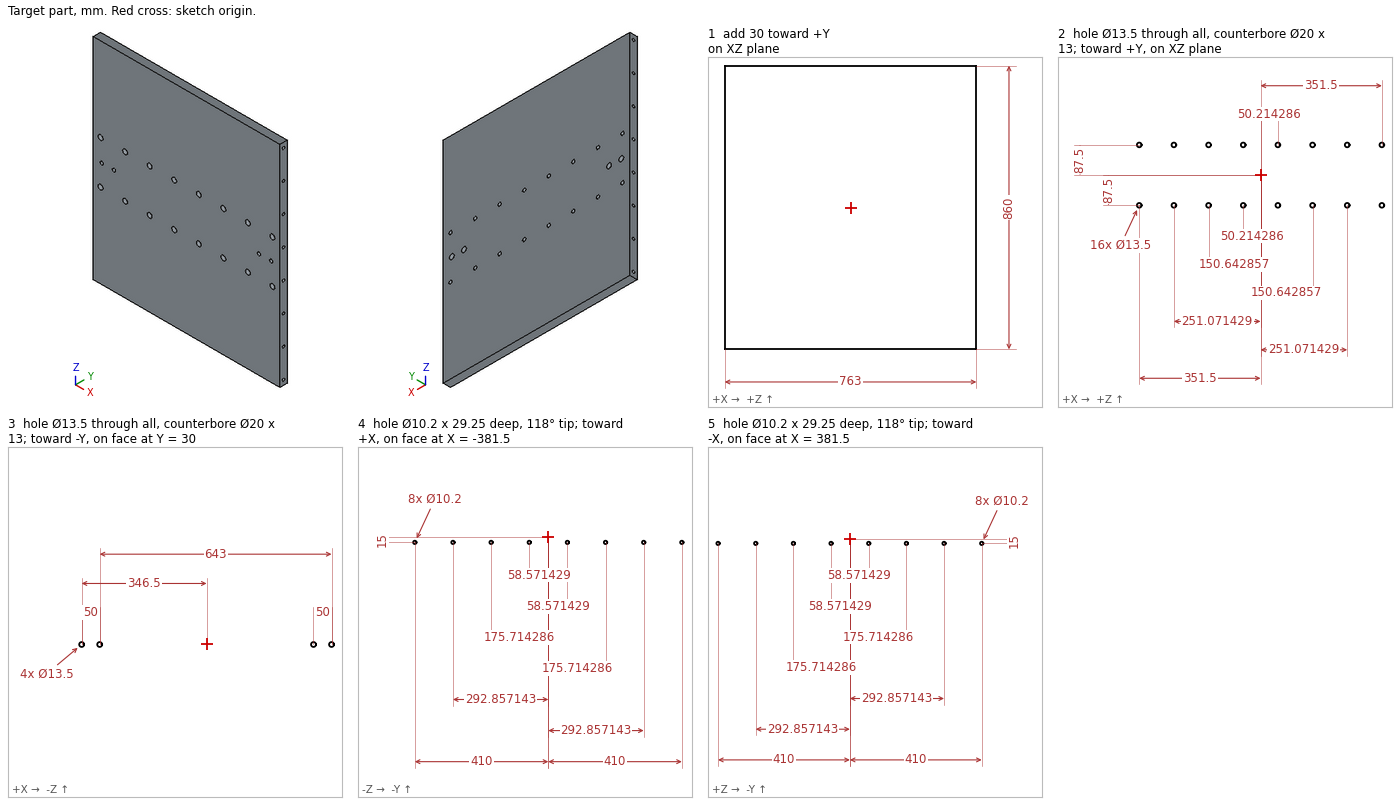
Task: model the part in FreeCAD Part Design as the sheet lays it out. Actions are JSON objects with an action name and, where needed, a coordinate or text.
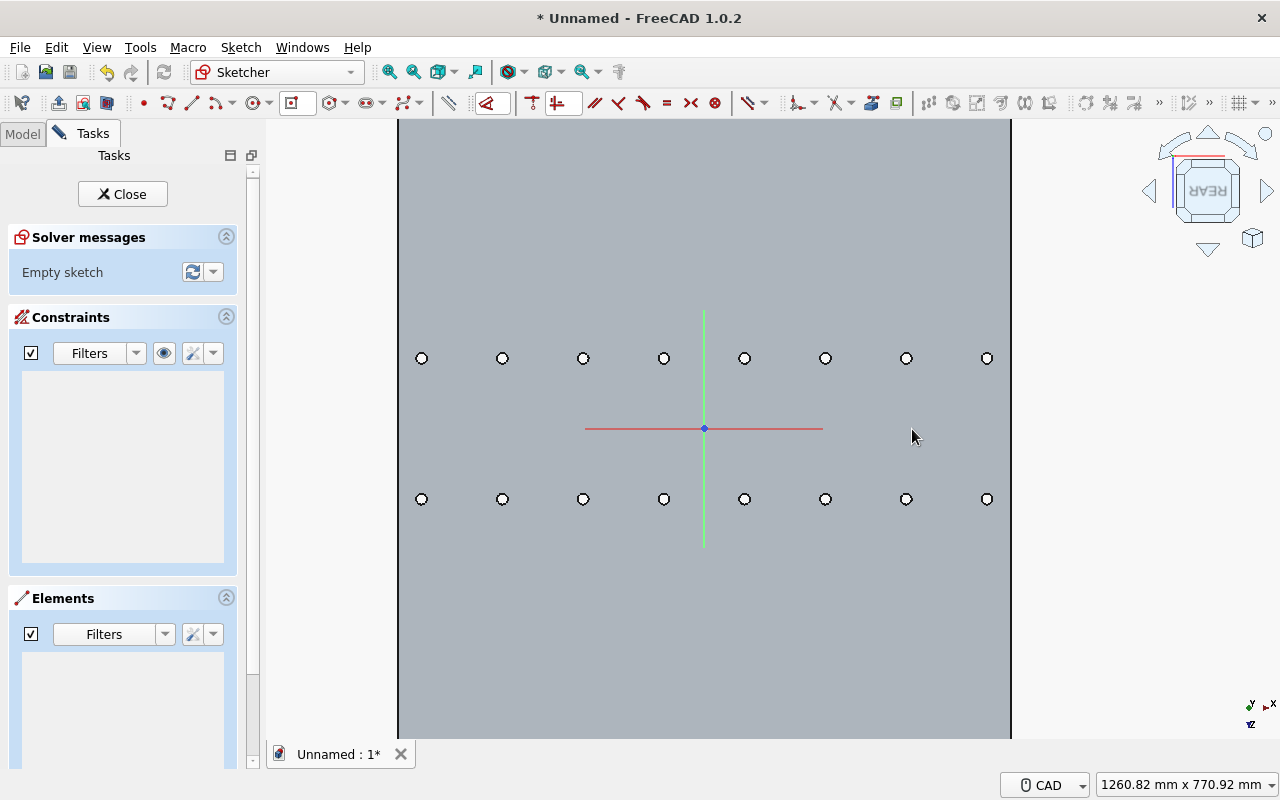
{"action": "left_click", "coordinate": [254, 104]}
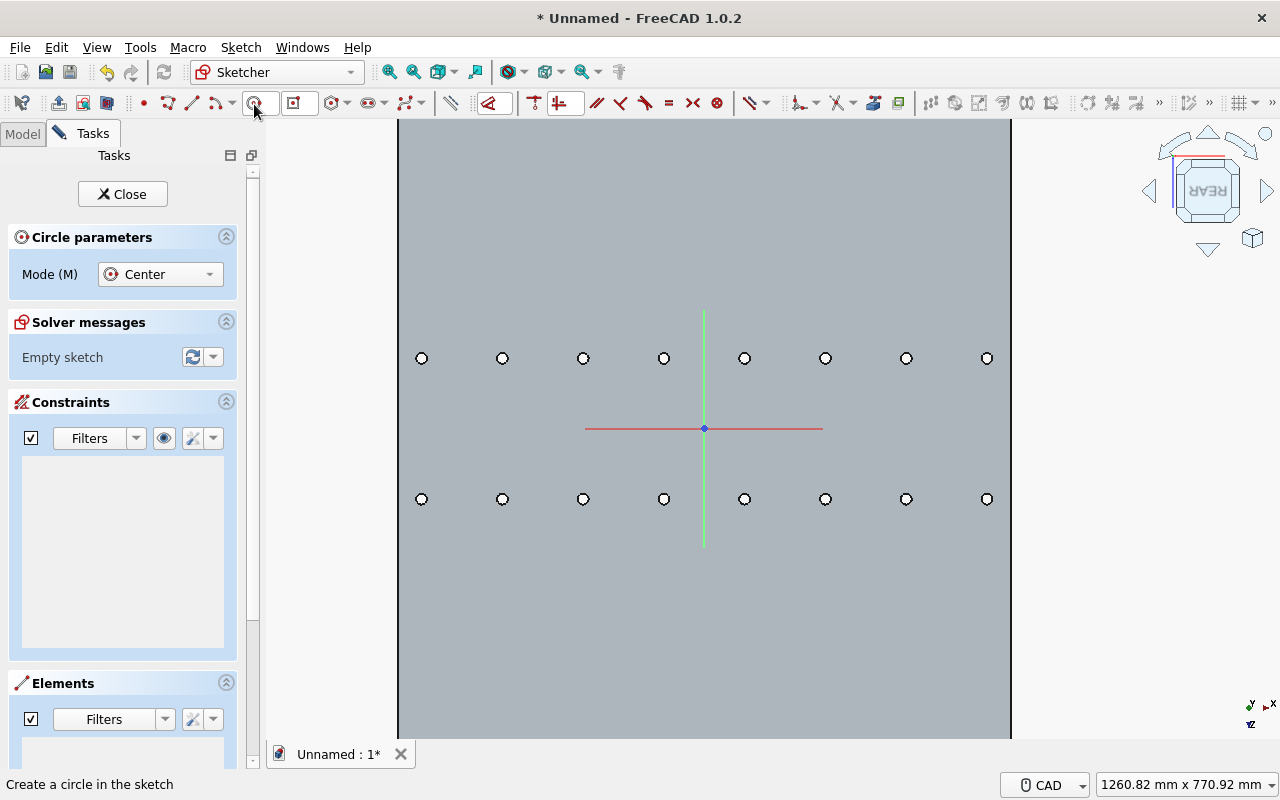
{"action": "scroll", "coordinate": [426, 429], "scroll_direction": "up", "scroll_amount": 8}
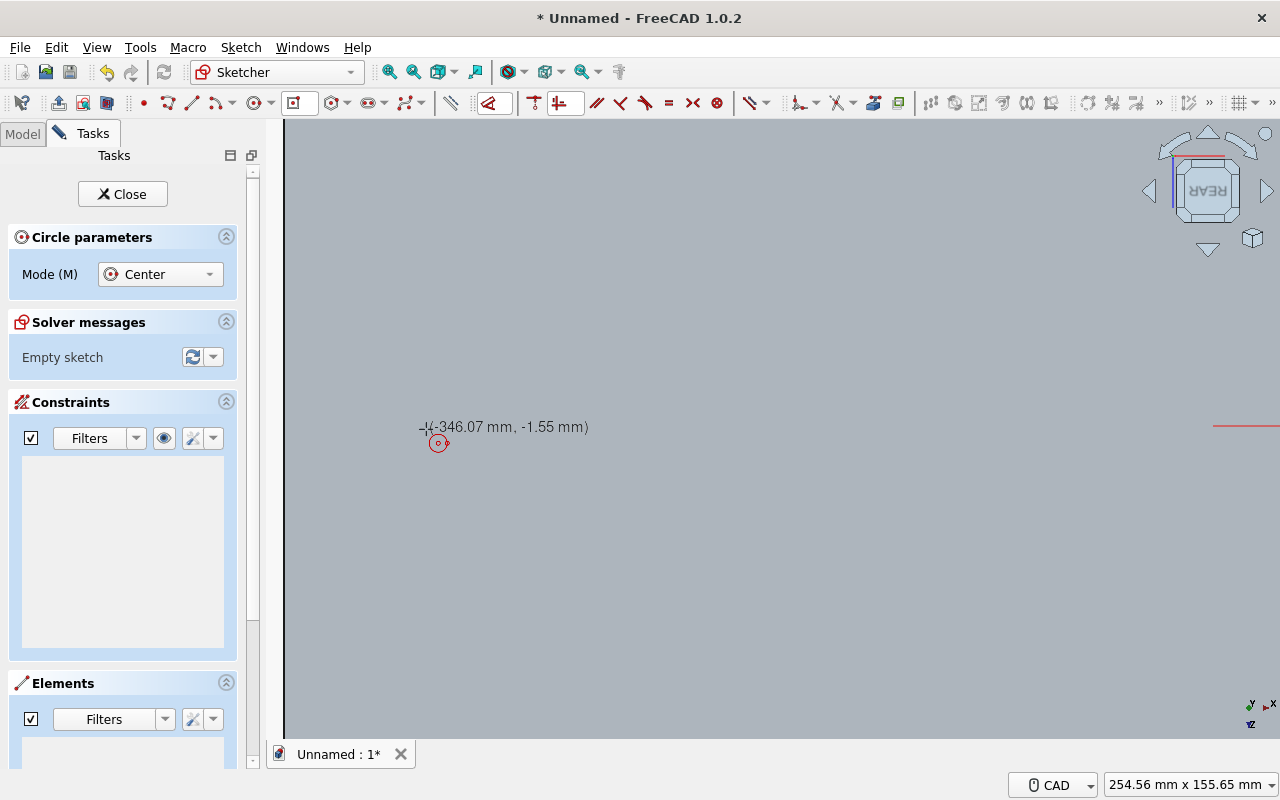
{"action": "scroll", "coordinate": [426, 430], "scroll_direction": "down", "scroll_amount": 8}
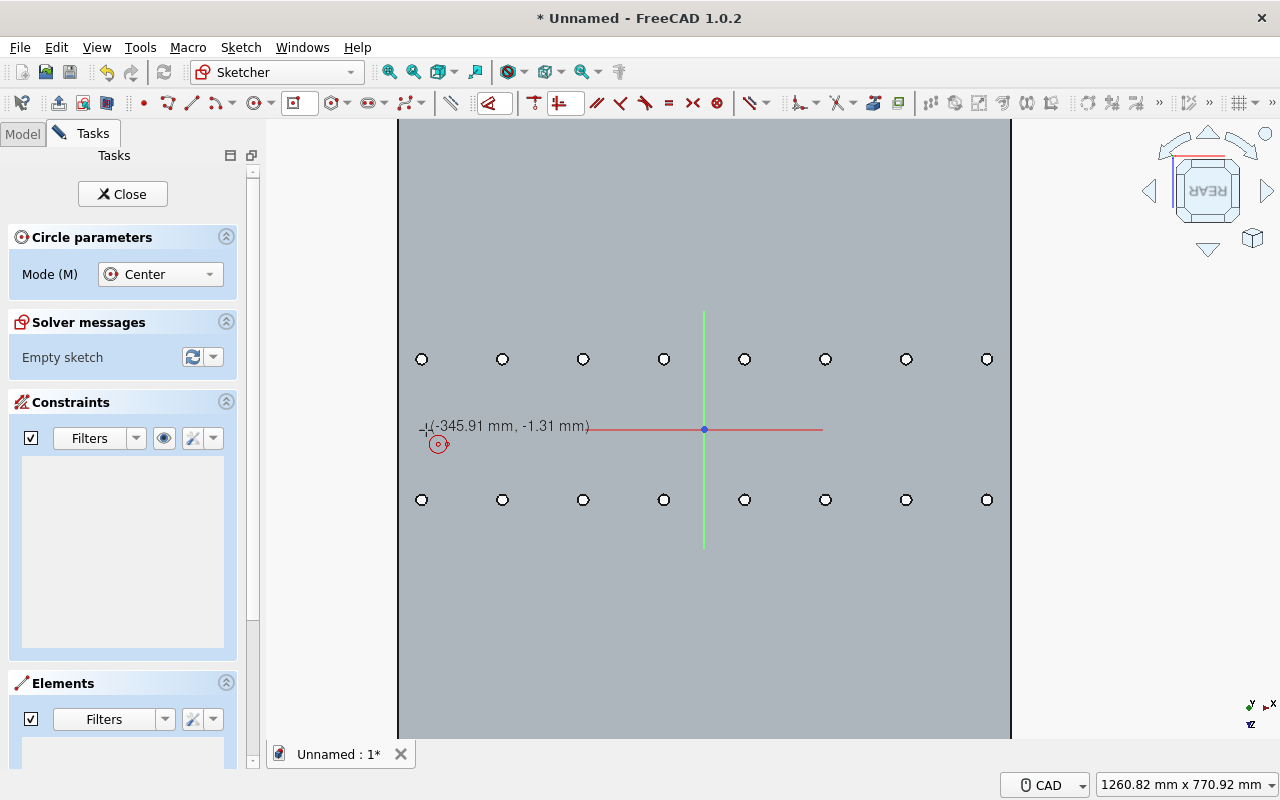
{"action": "left_click", "coordinate": [426, 430]}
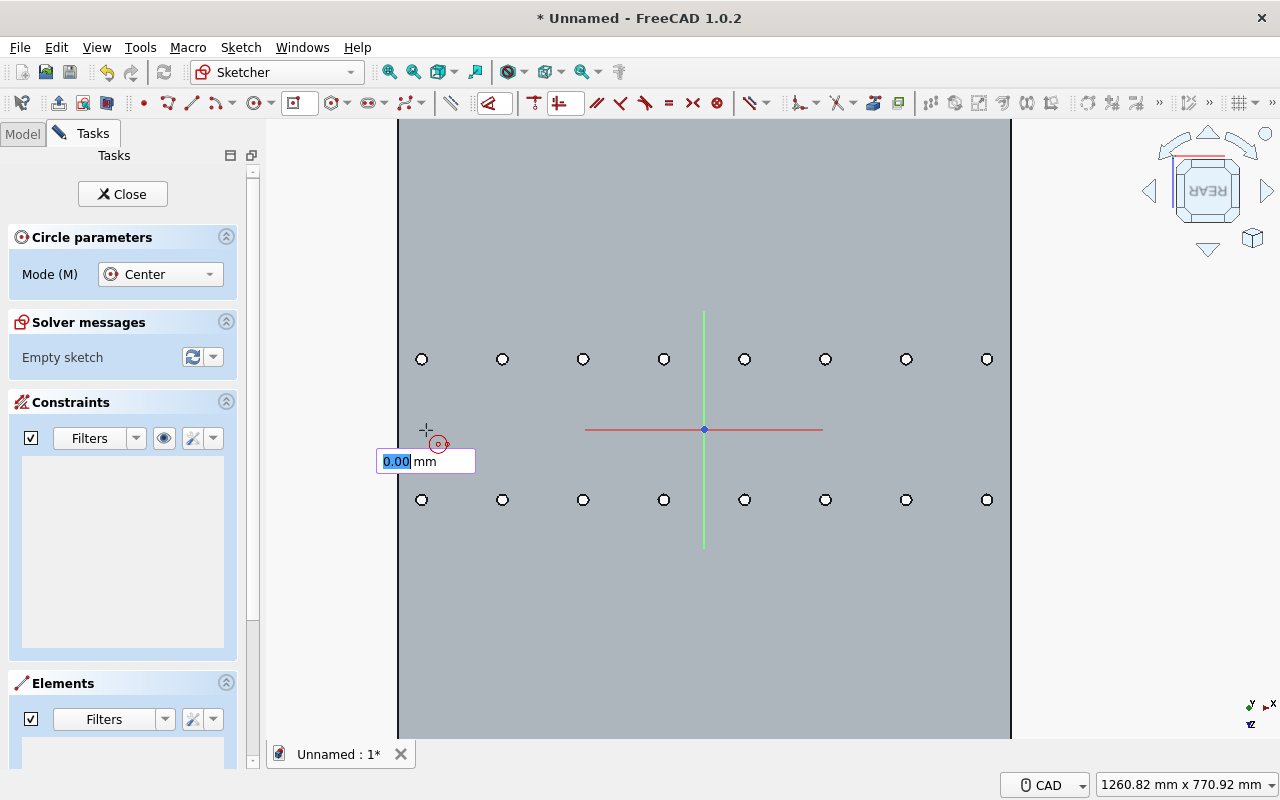
{"action": "scroll", "coordinate": [424, 435], "scroll_direction": "up", "scroll_amount": 6}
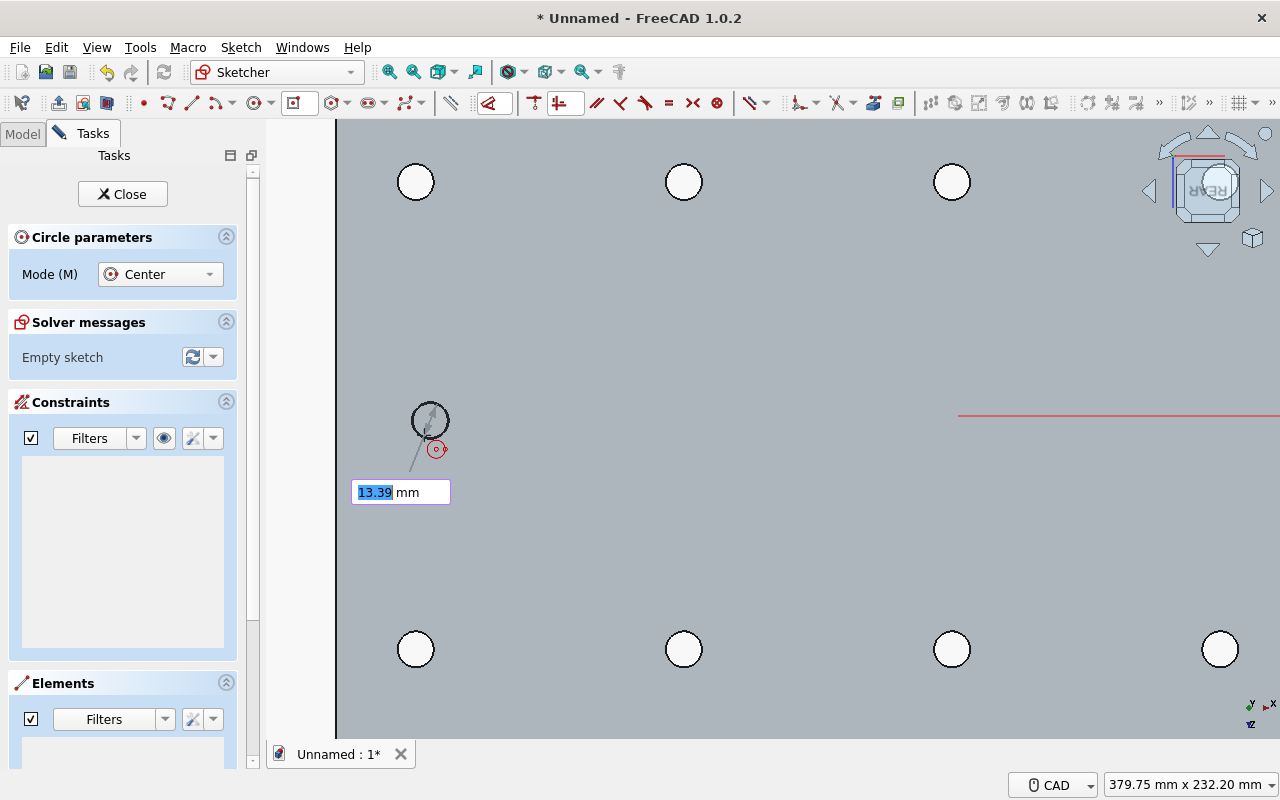
{"action": "left_click", "coordinate": [423, 433]}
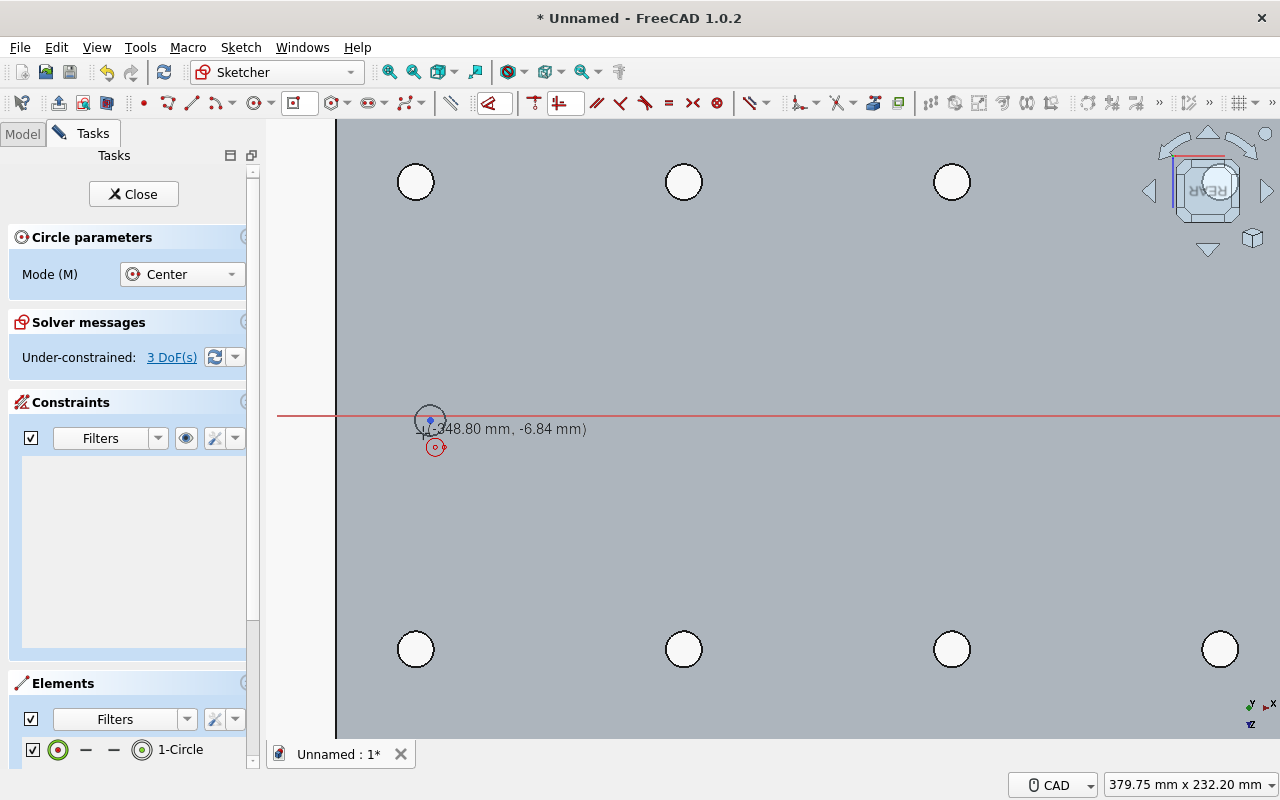
{"action": "scroll", "coordinate": [563, 416], "scroll_direction": "up", "scroll_amount": 2}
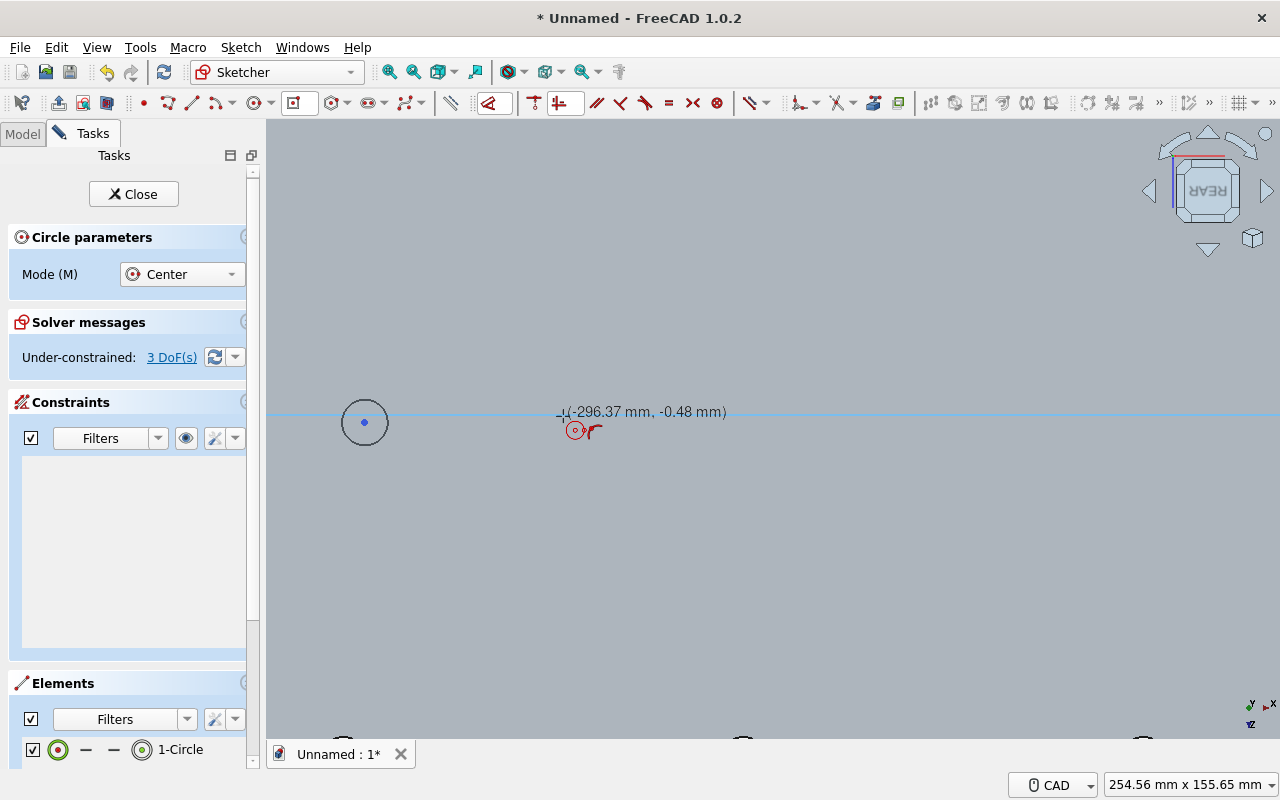
{"action": "scroll", "coordinate": [442, 432], "scroll_direction": "down", "scroll_amount": 8}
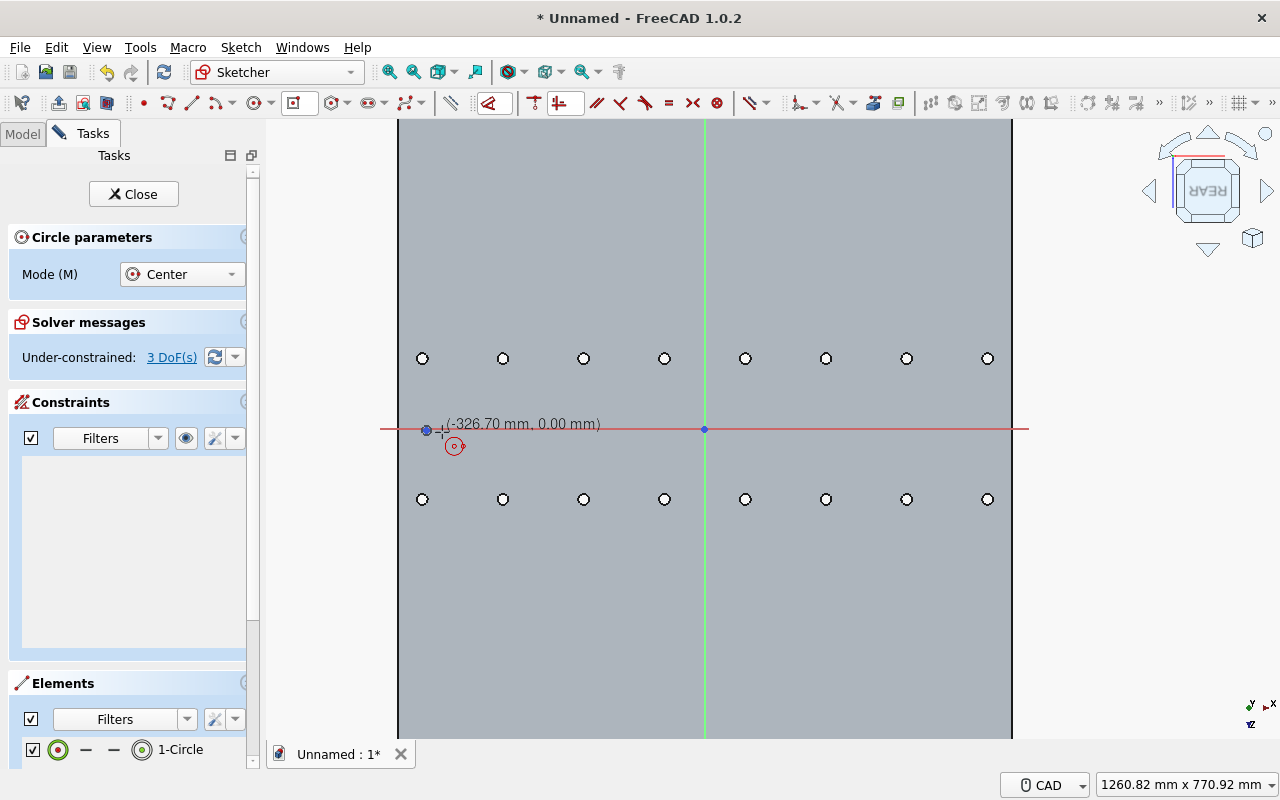
{"action": "left_click", "coordinate": [466, 429]}